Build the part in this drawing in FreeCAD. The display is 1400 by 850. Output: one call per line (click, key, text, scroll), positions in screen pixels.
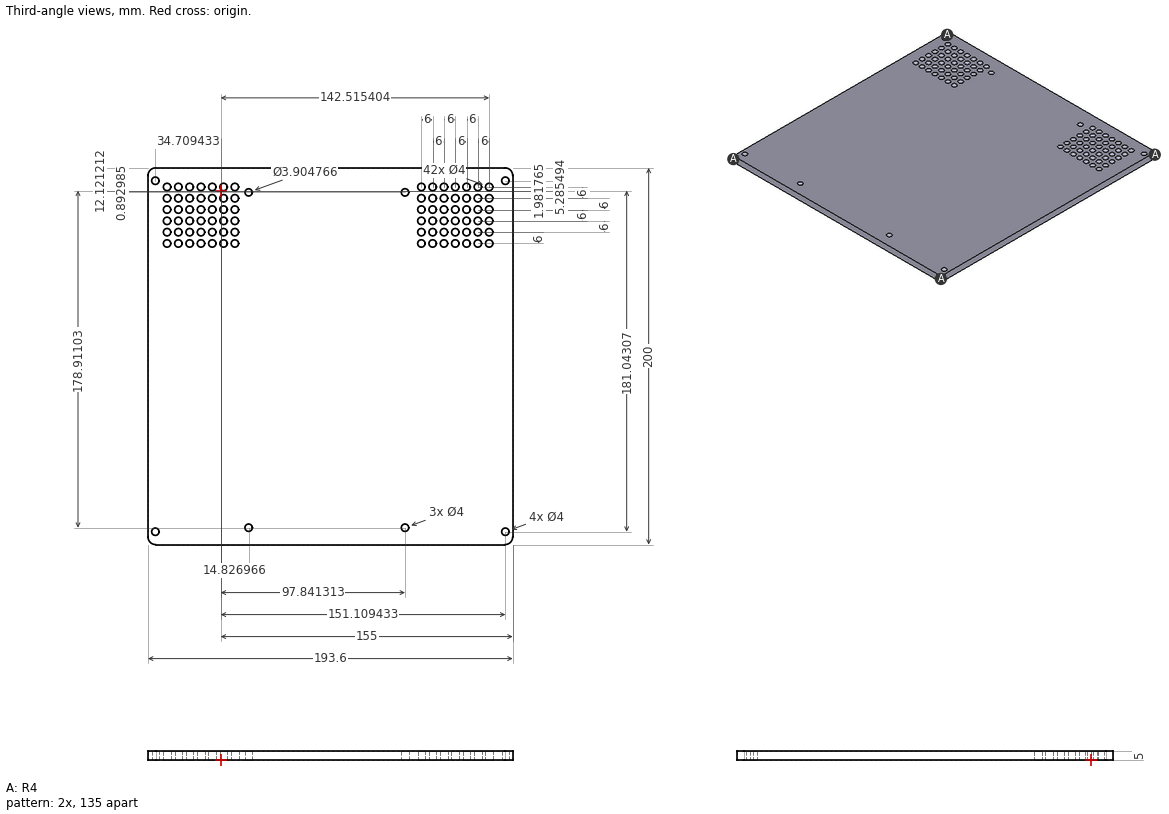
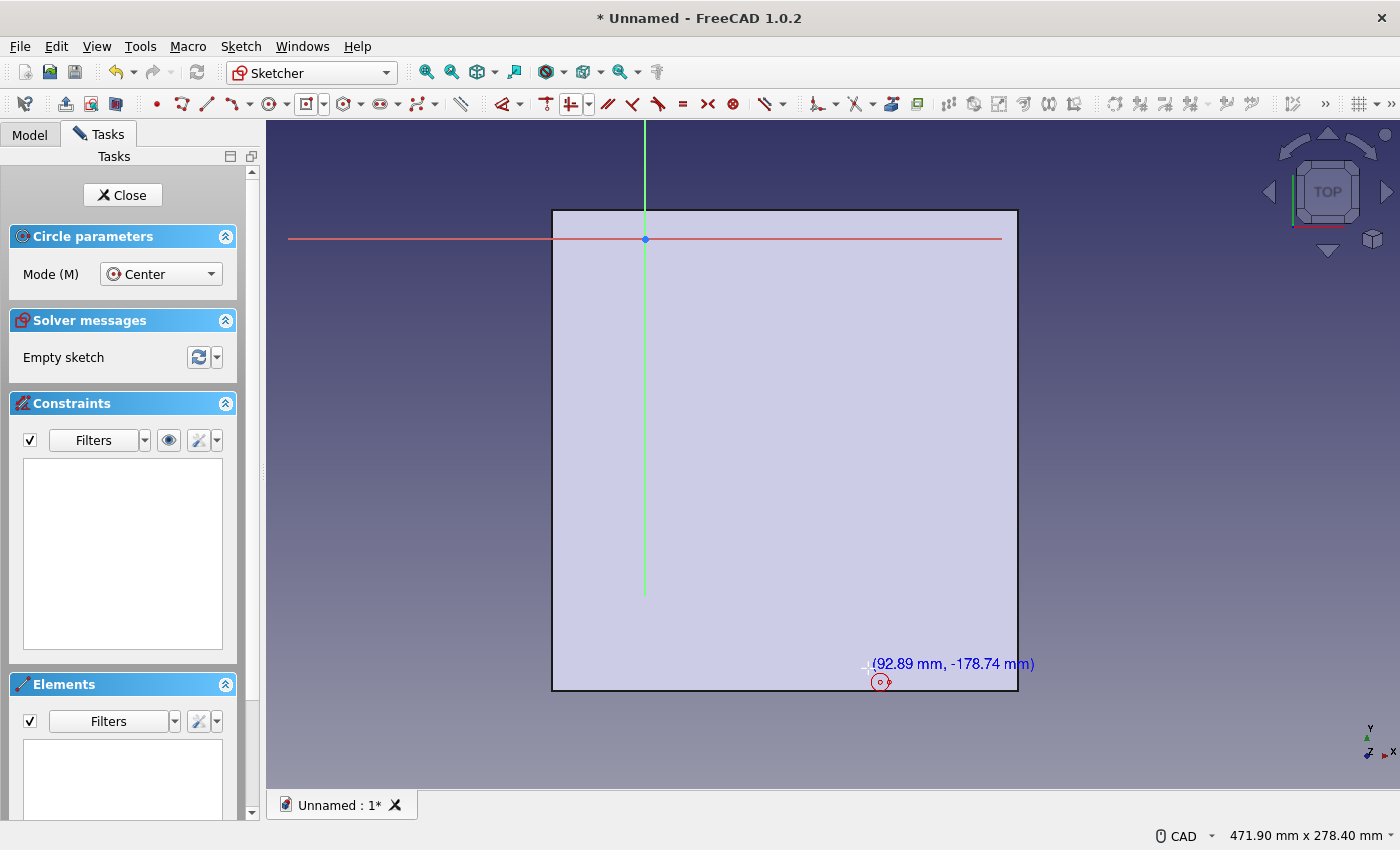
click(880, 669)
move(884, 666)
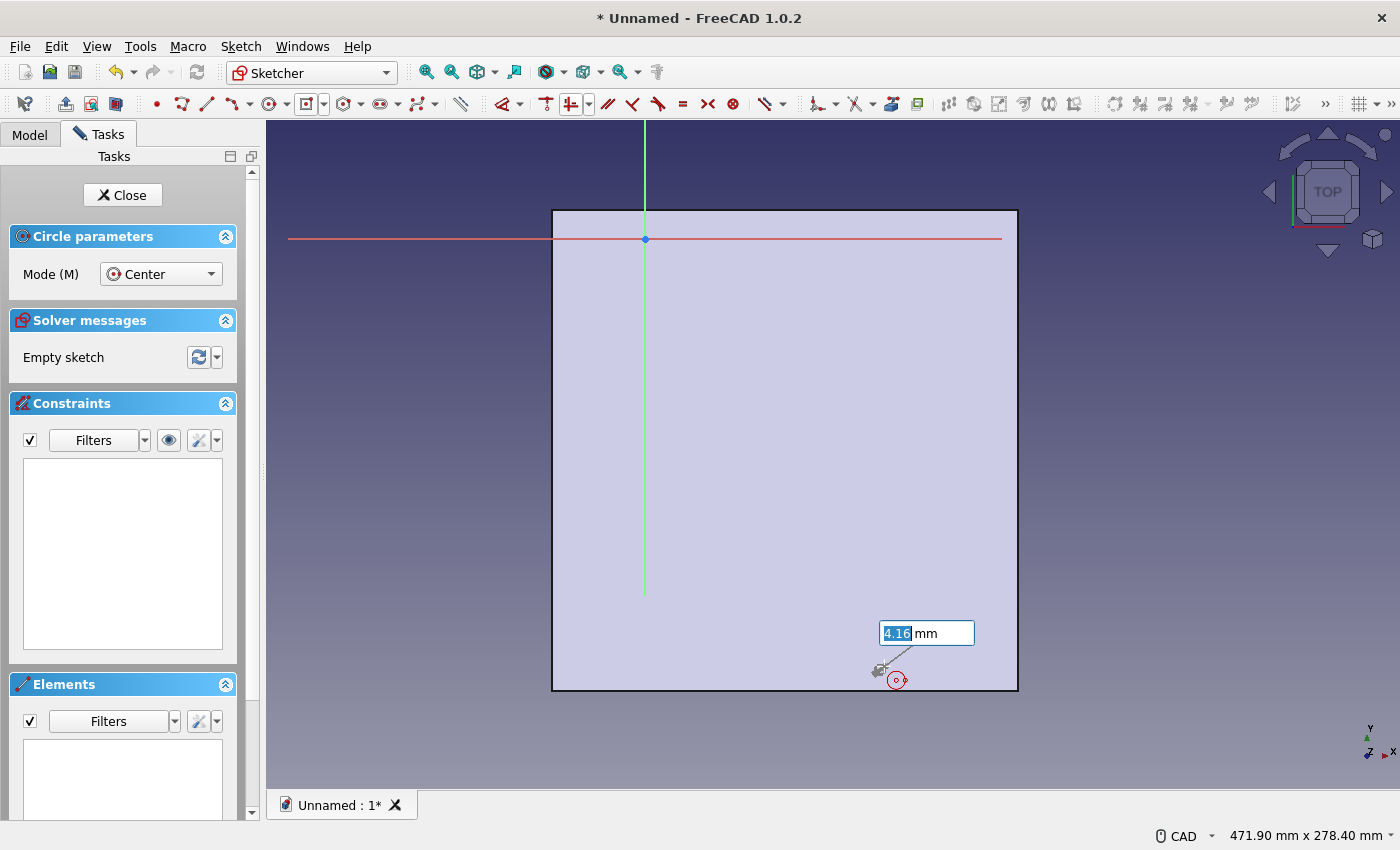
text(4)
key(Return)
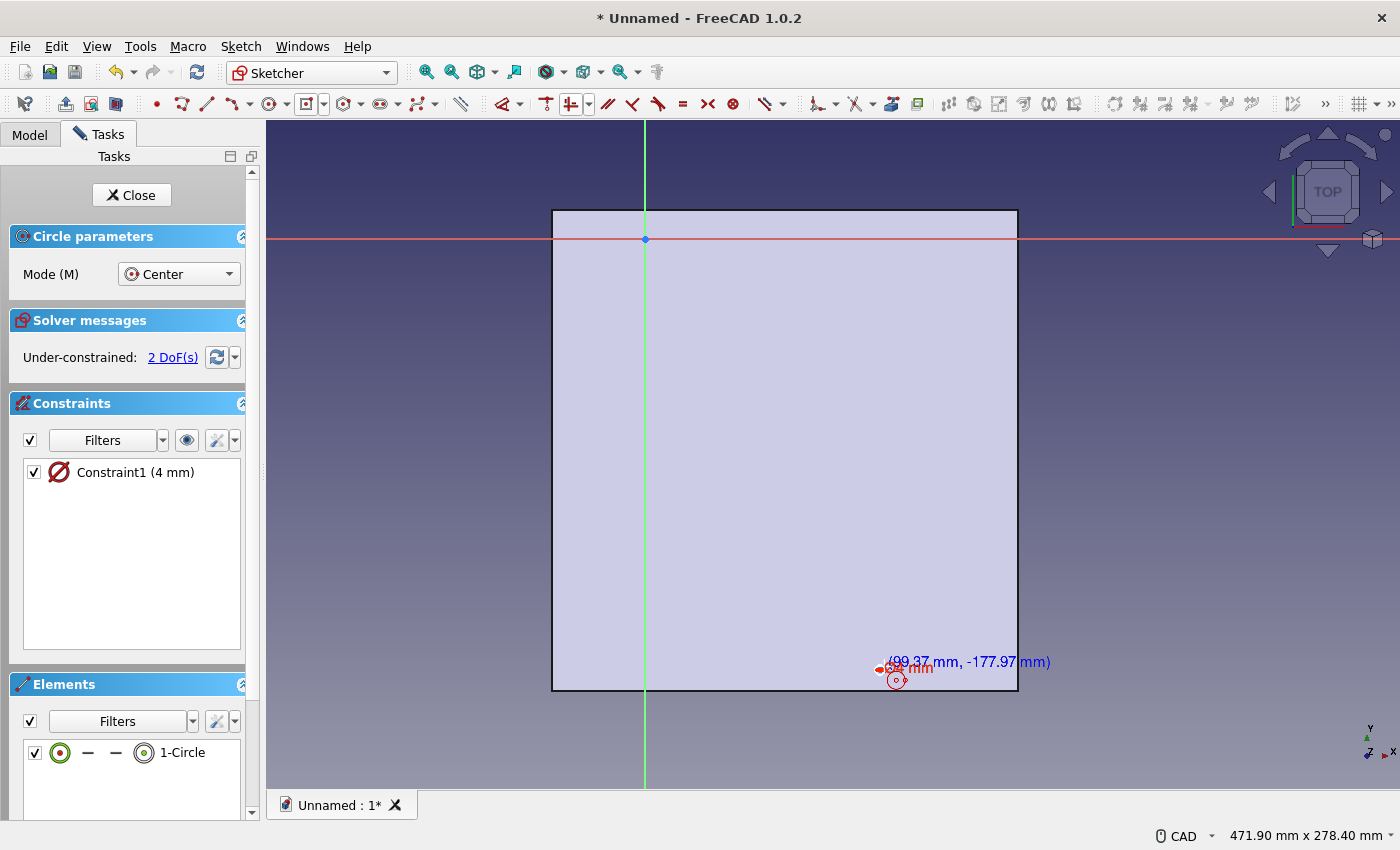
scroll(880, 241, up, 11)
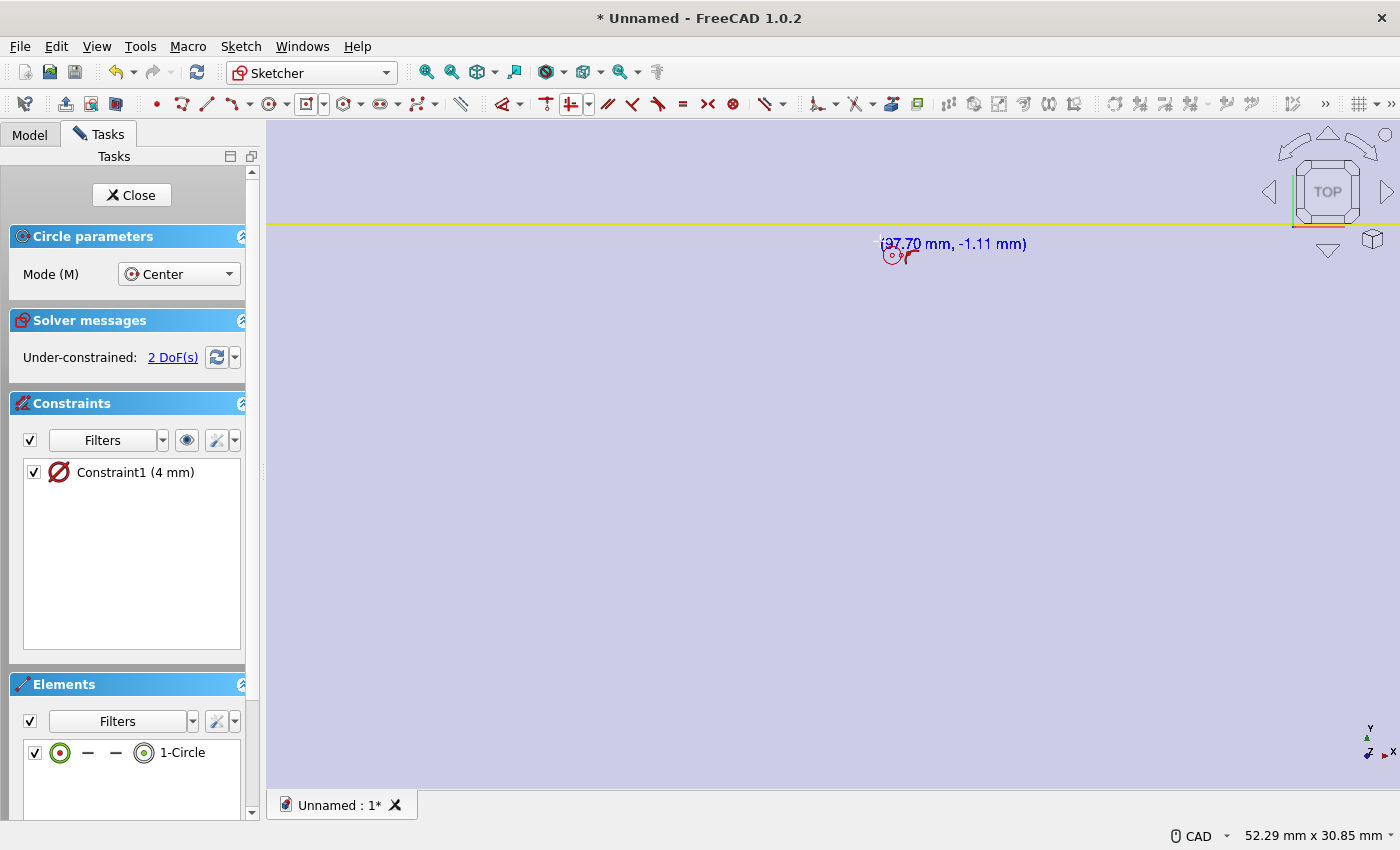
click(879, 244)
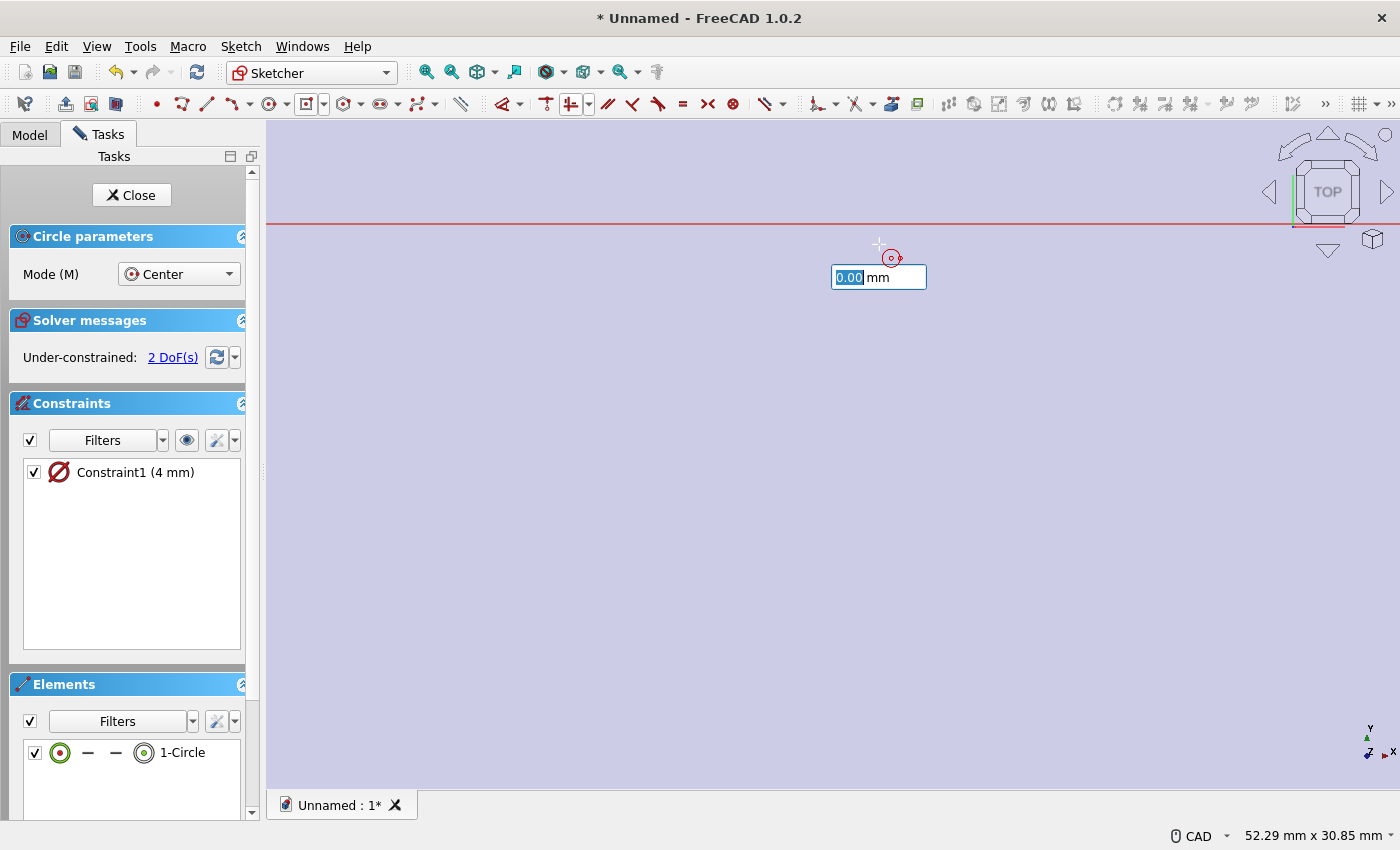
scroll(880, 240, down, 11)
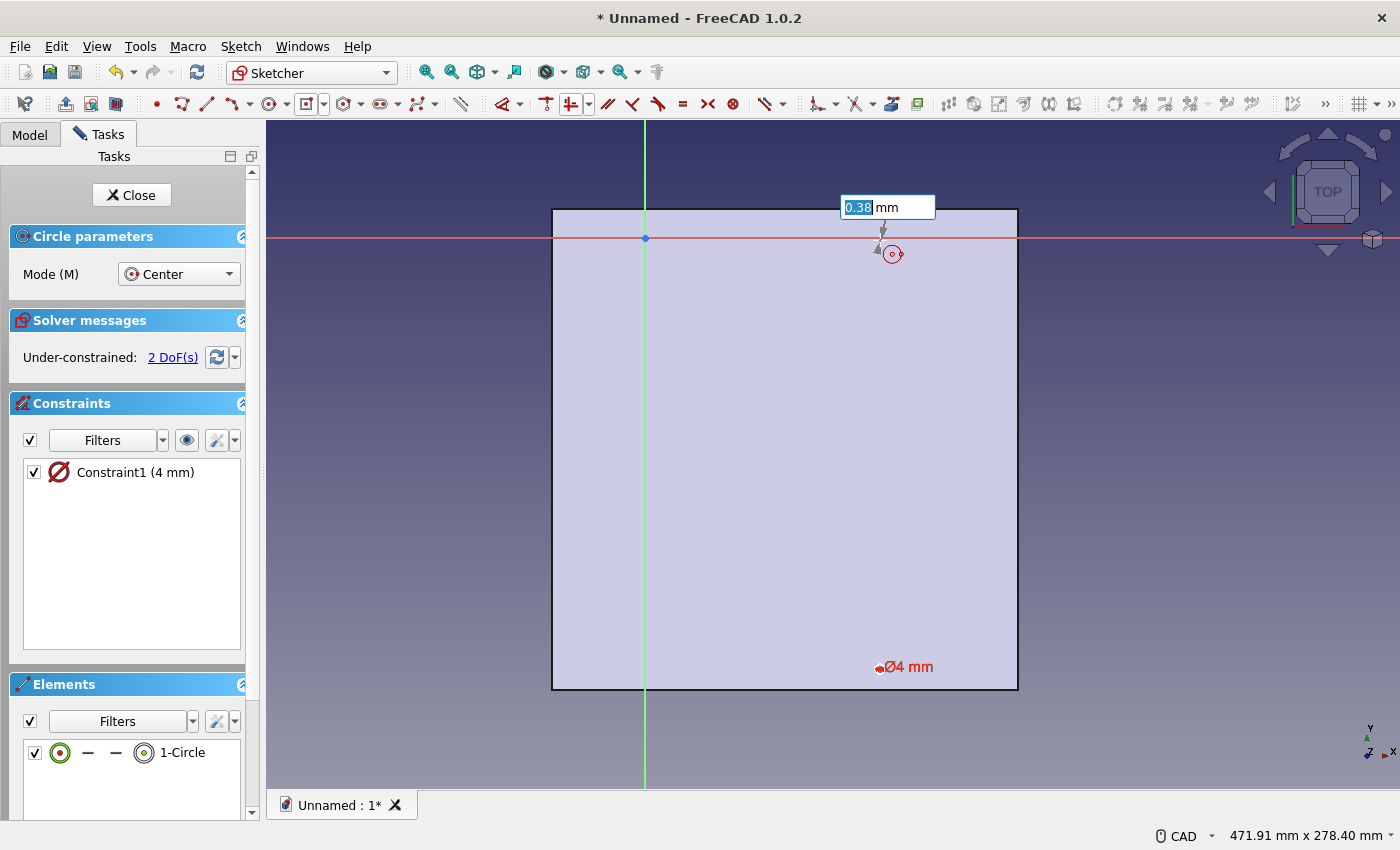
scroll(884, 244, up, 6)
move(882, 244)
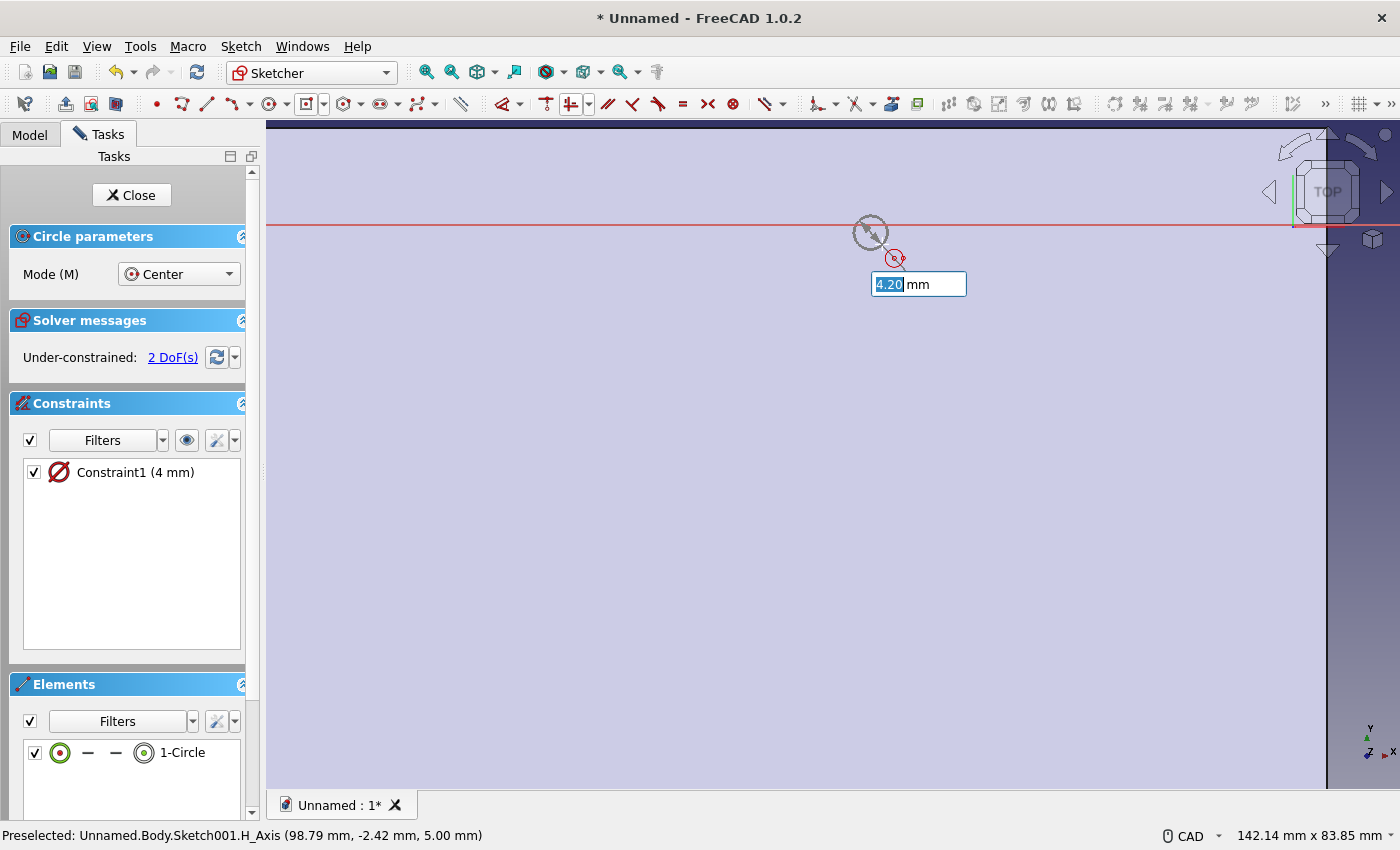
text(4)
key(Return)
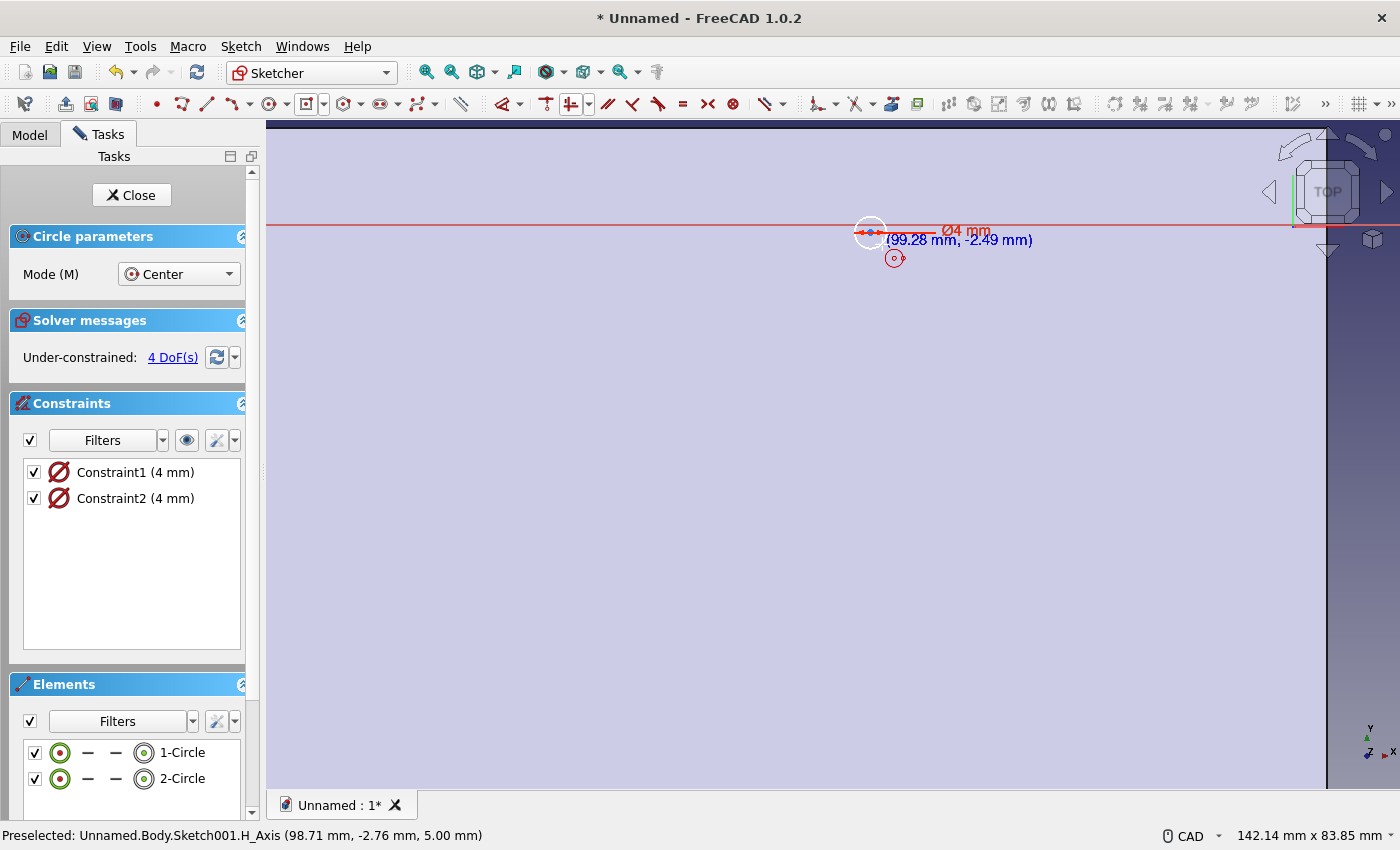
scroll(884, 244, down, 6)